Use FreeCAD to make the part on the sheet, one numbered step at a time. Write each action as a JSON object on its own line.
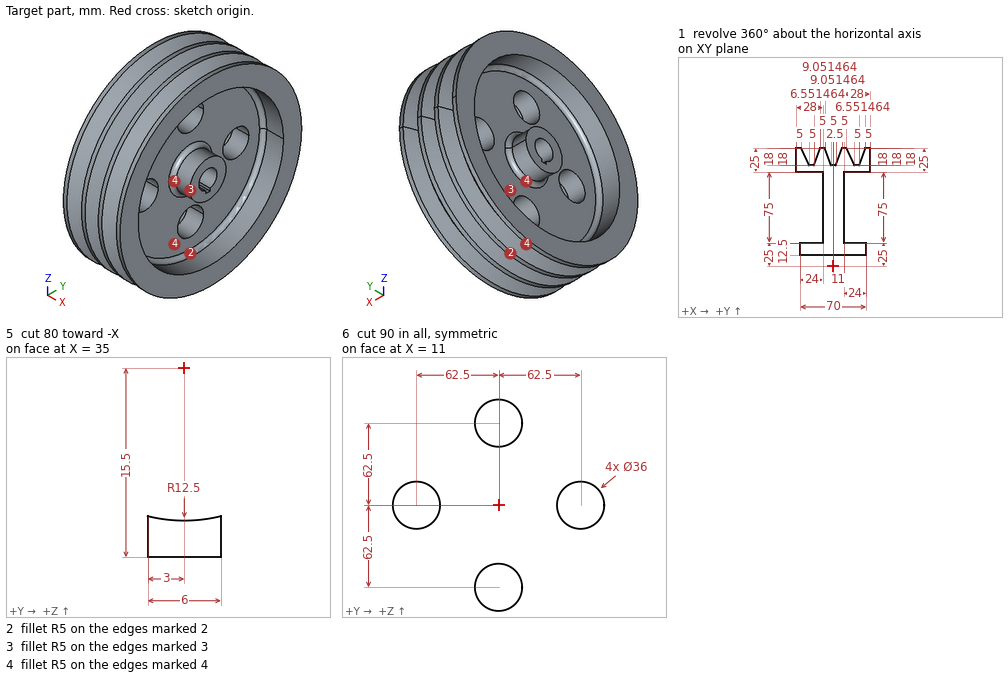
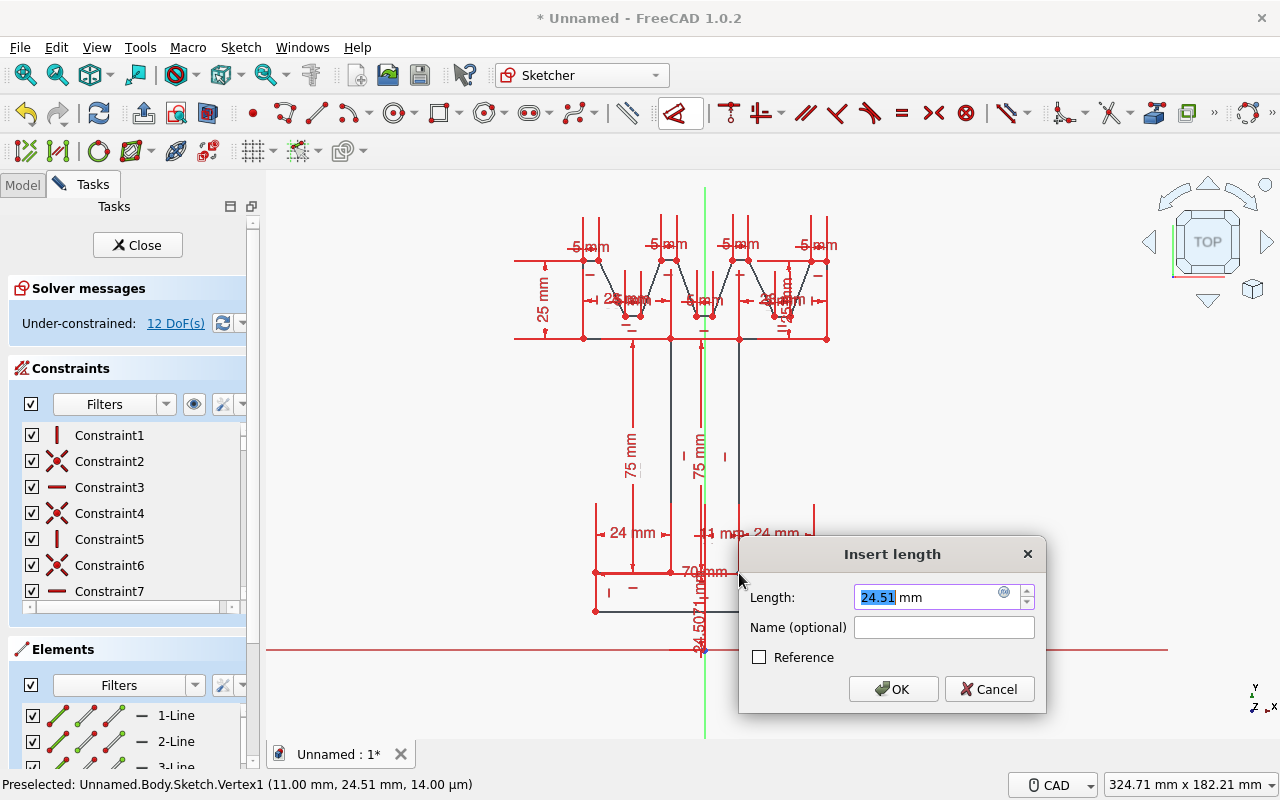
{"action": "type", "text": "25"}
{"action": "key", "text": "Return"}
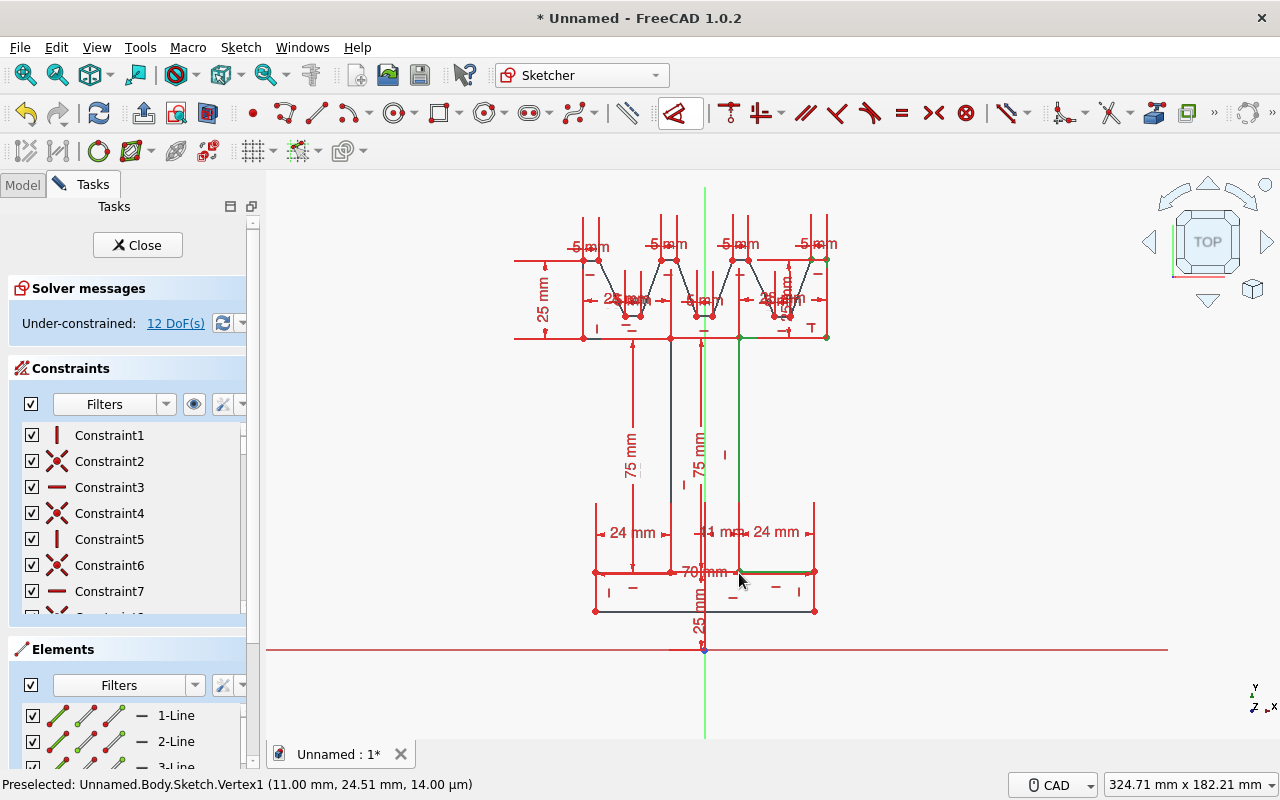
{"action": "left_click", "coordinate": [671, 573]}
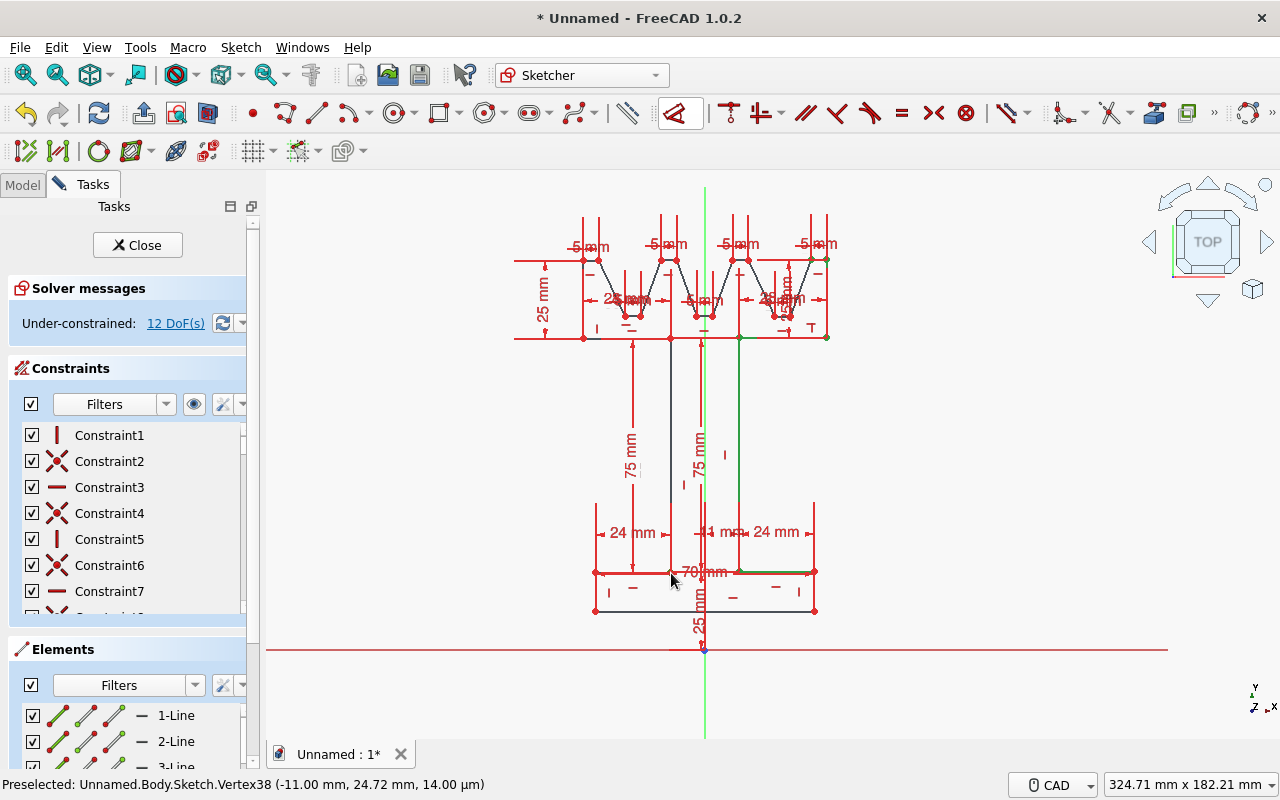
{"action": "key", "text": "i"}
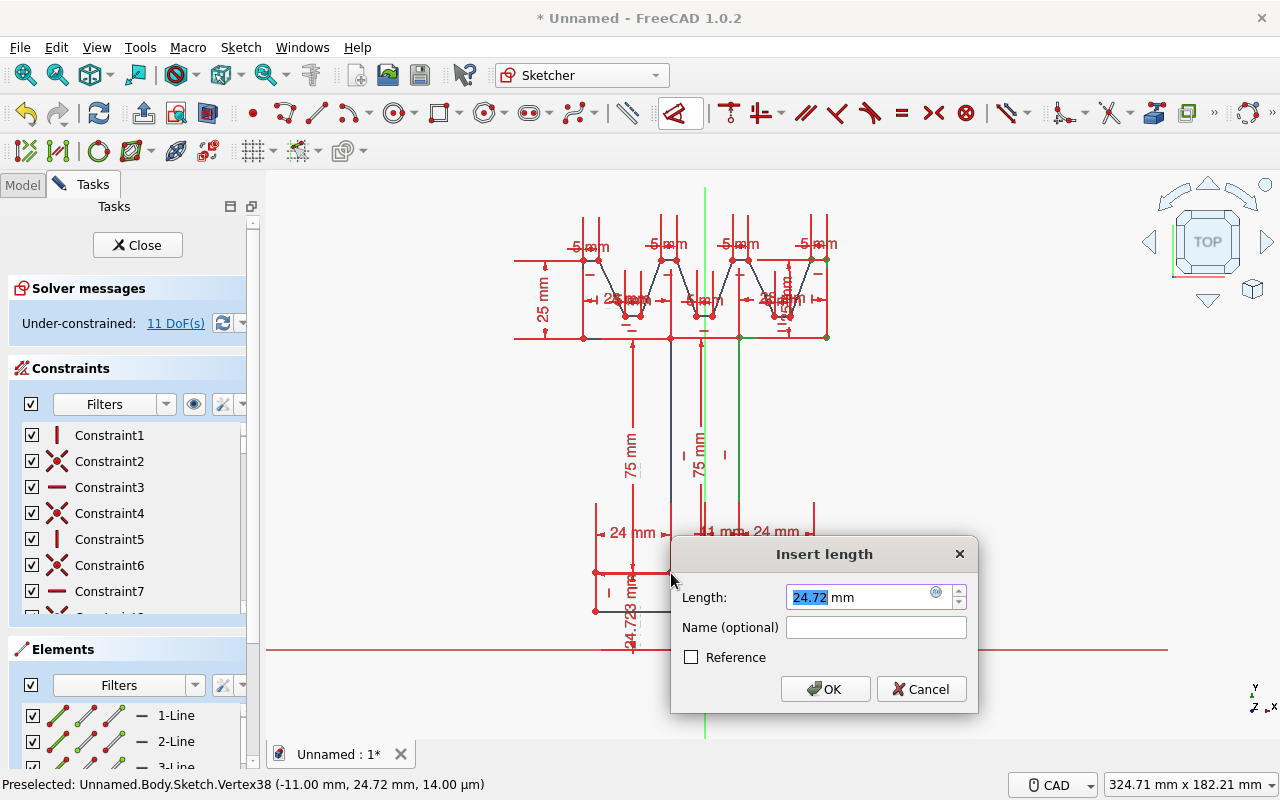
{"action": "type", "text": "25"}
{"action": "key", "text": "Return"}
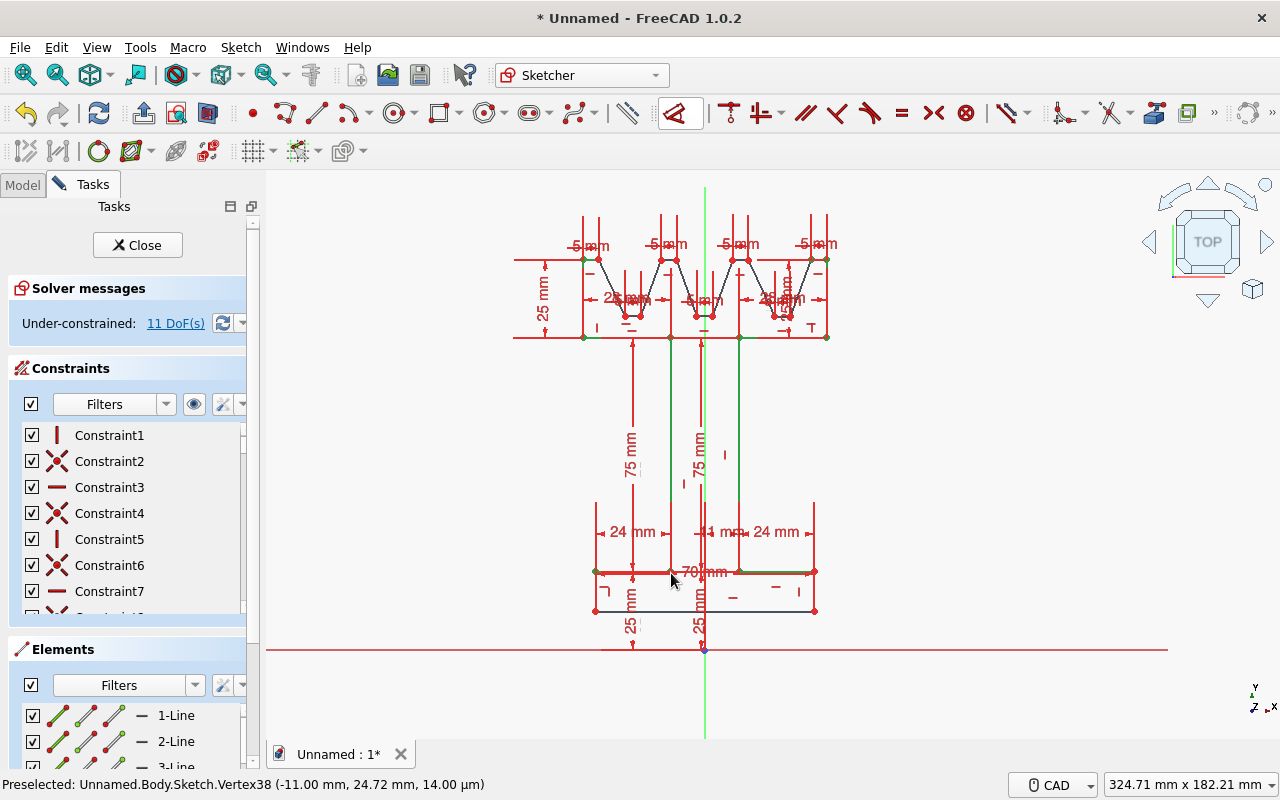
{"action": "left_click", "coordinate": [805, 277]}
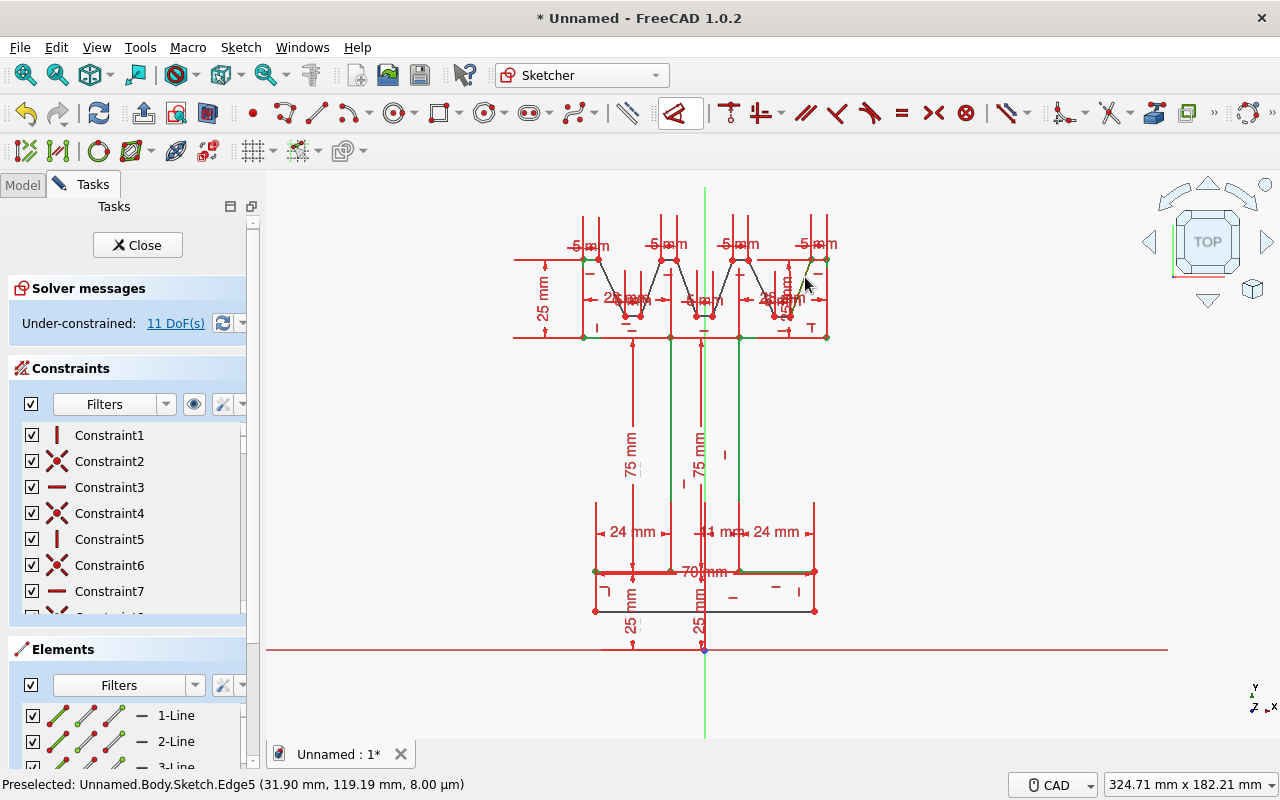
{"action": "left_click", "coordinate": [698, 114]}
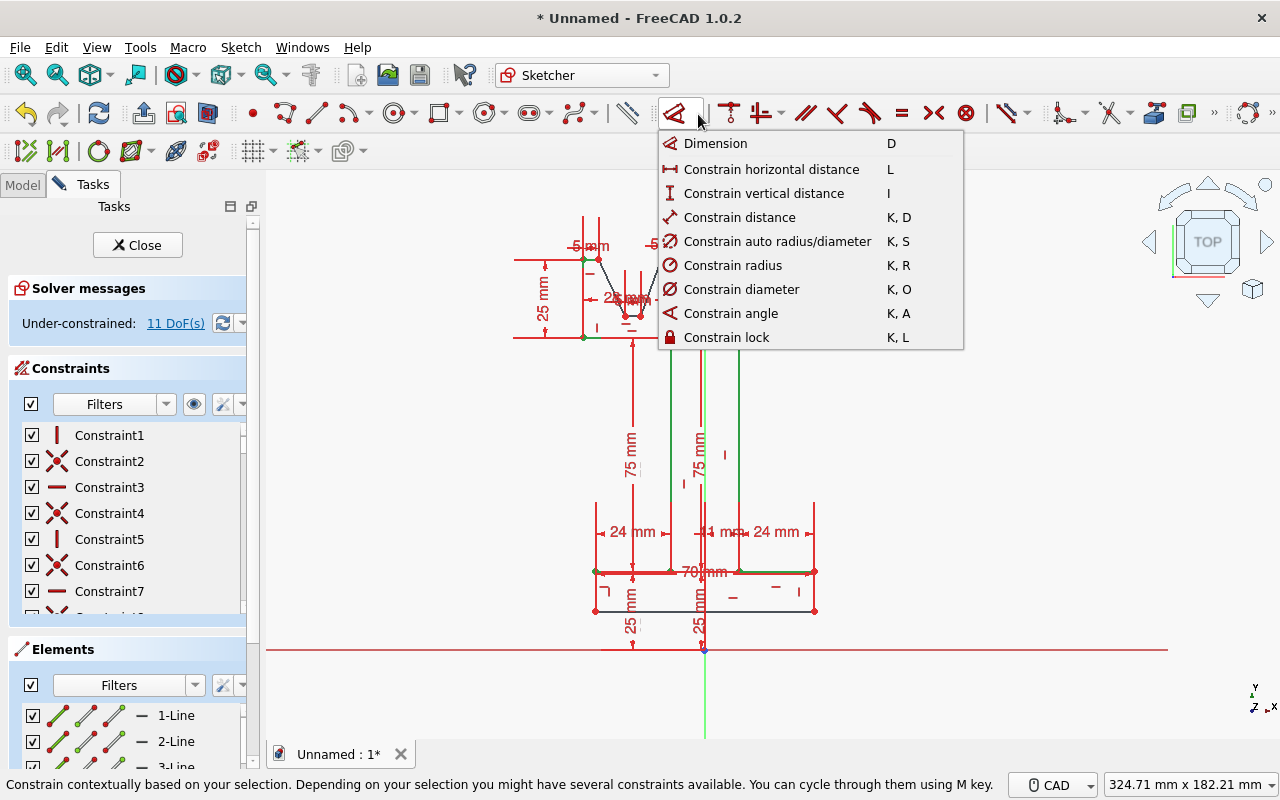
{"action": "left_click", "coordinate": [811, 193]}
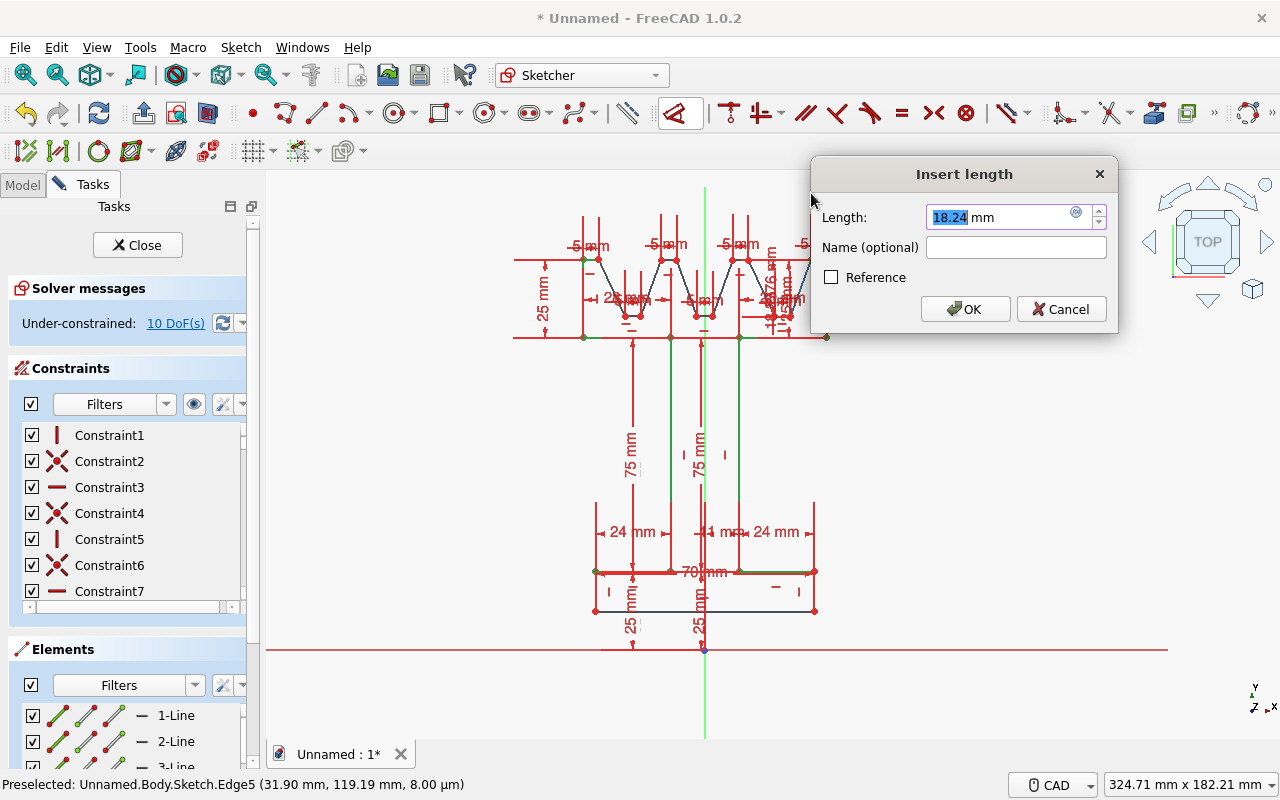
{"action": "type", "text": "18"}
{"action": "key", "text": "Return"}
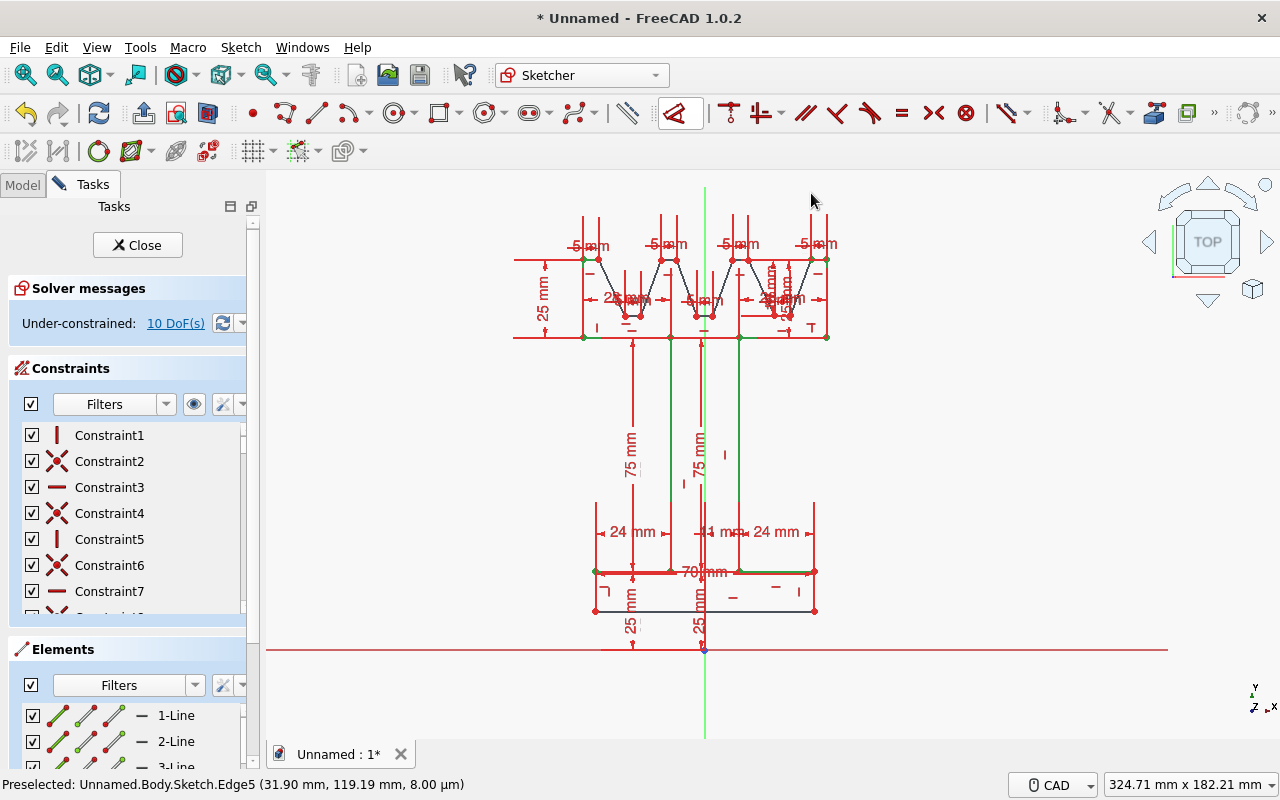
{"action": "left_click", "coordinate": [756, 277]}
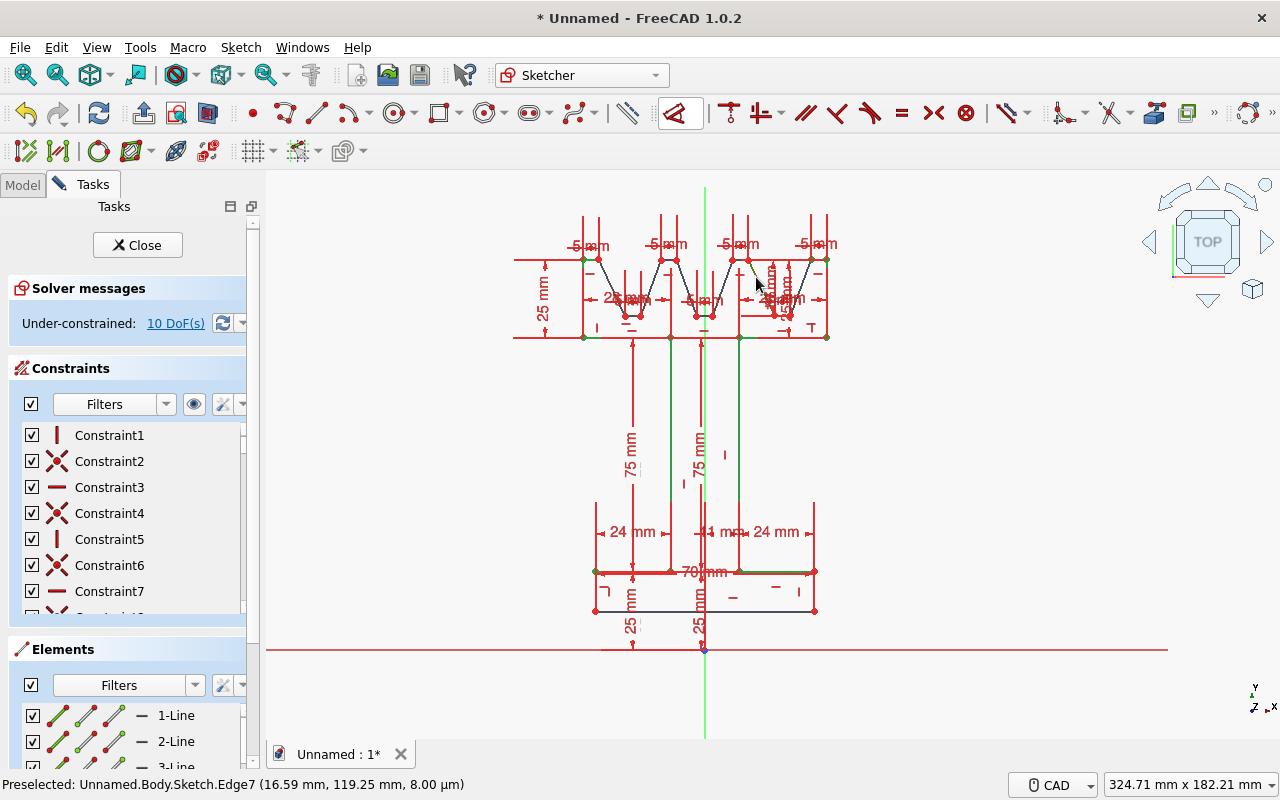
{"action": "left_click", "coordinate": [698, 114]}